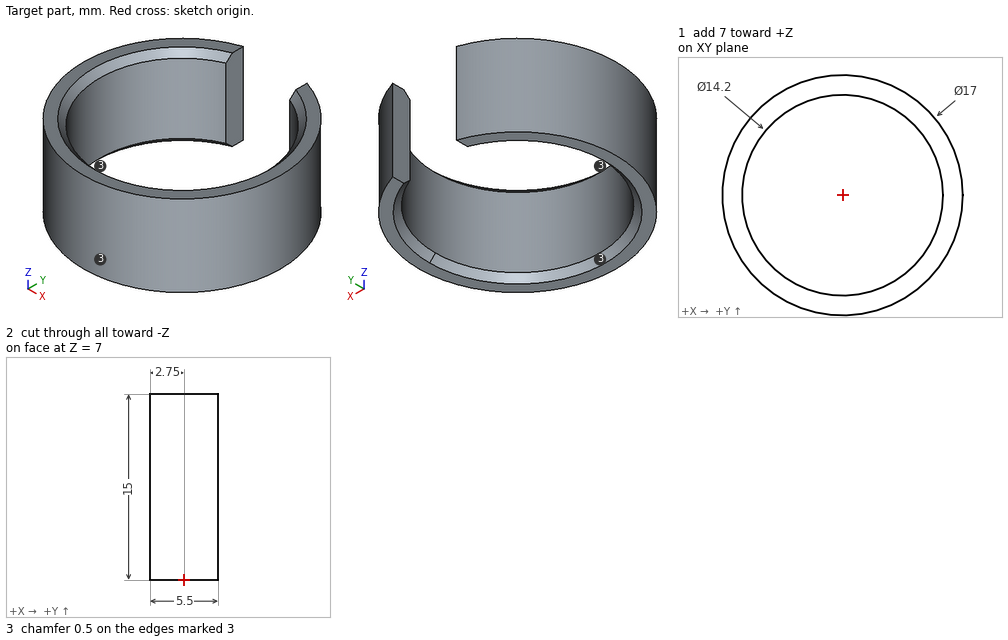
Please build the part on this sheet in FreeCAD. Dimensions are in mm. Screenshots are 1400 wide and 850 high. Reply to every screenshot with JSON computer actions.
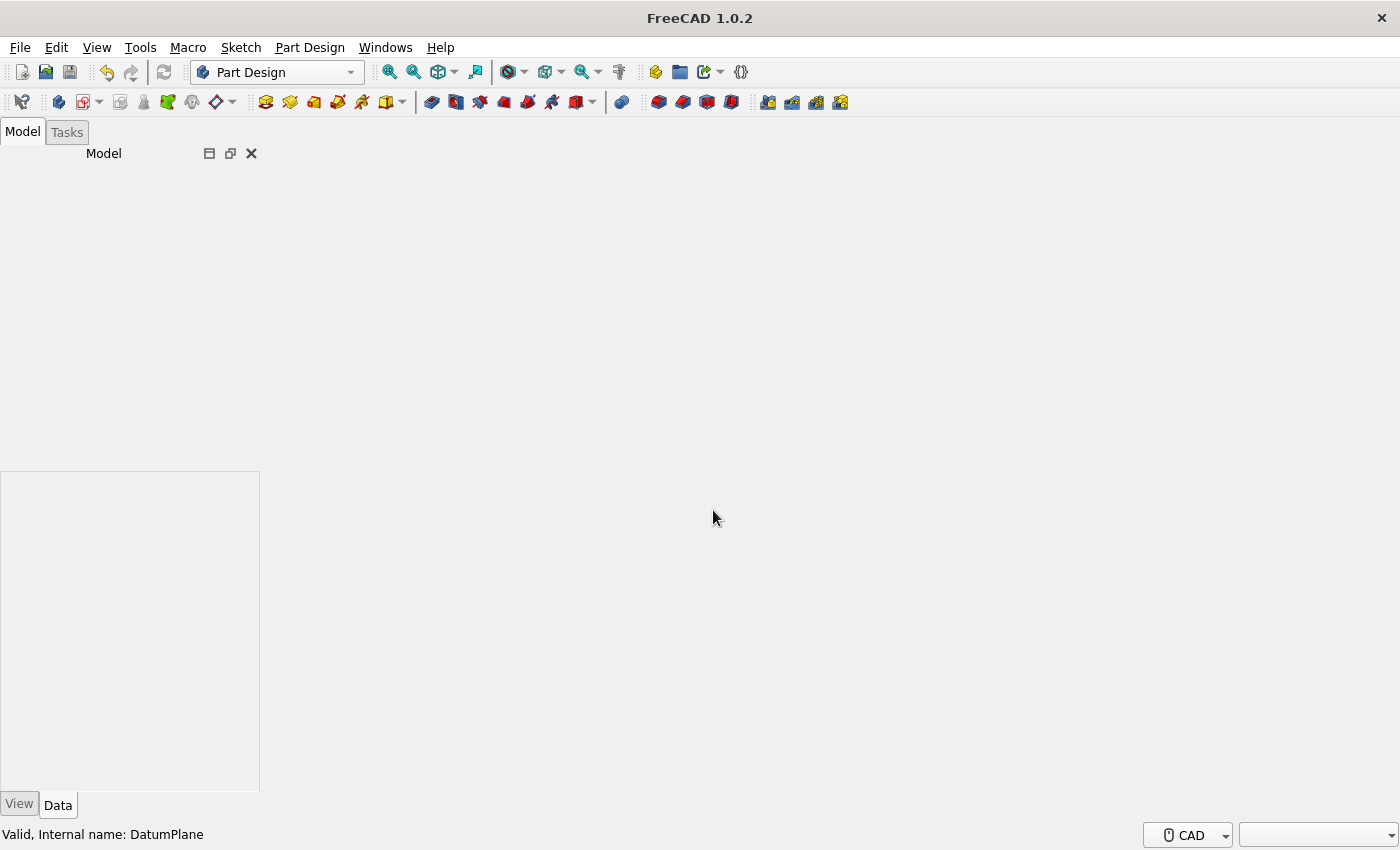
{"action": "left_click", "coordinate": [22, 72]}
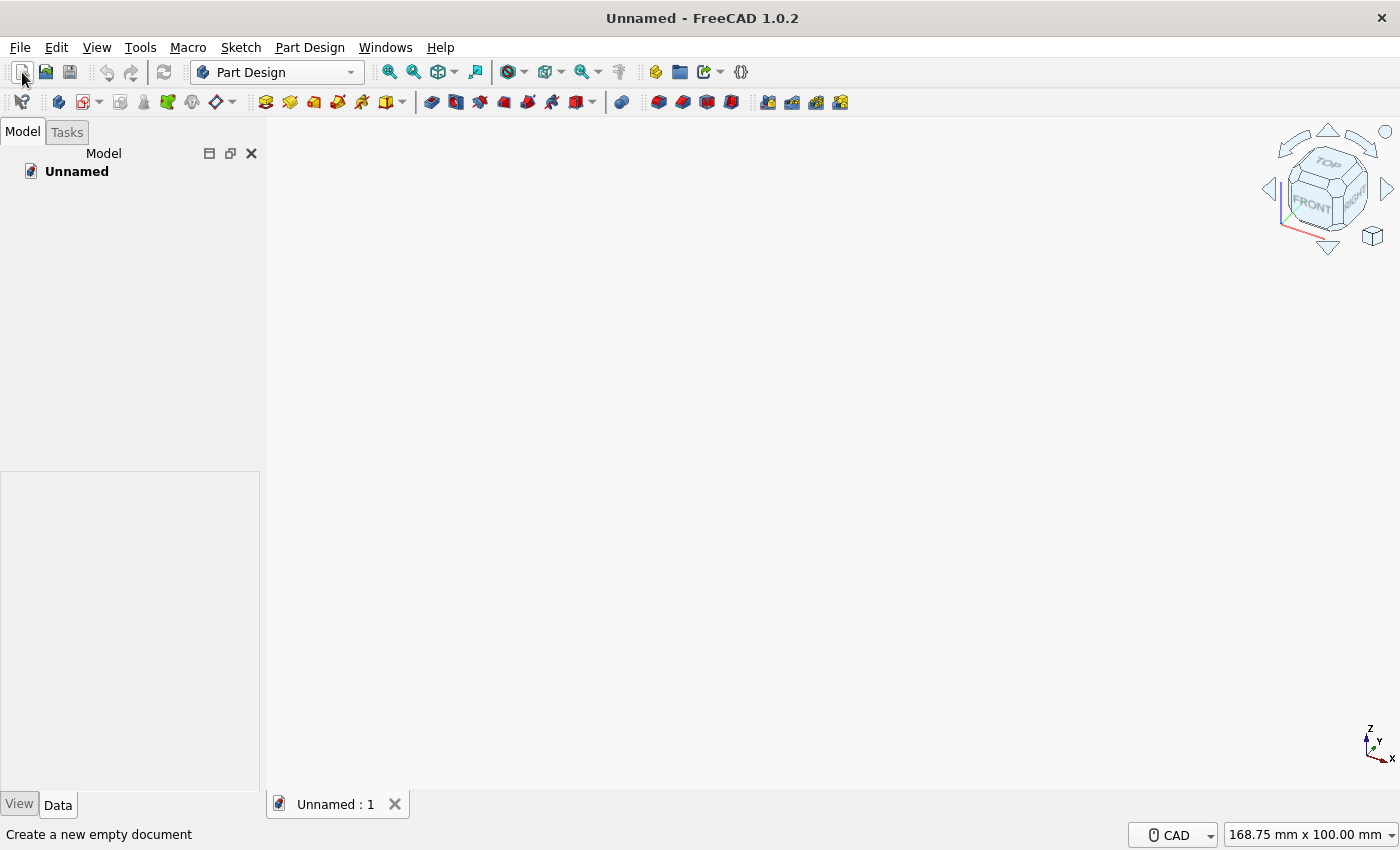
{"action": "left_click", "coordinate": [84, 102]}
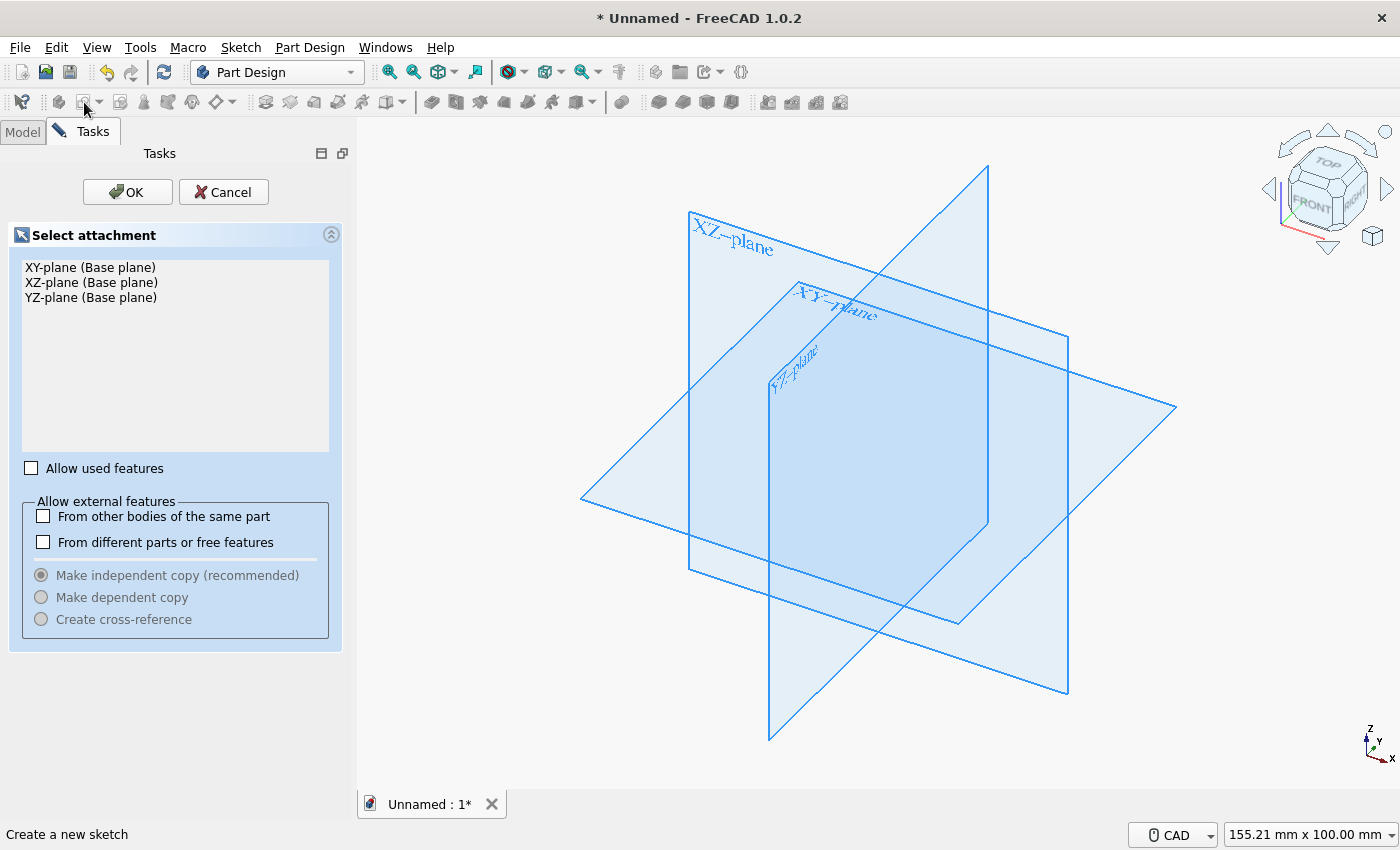
{"action": "left_click", "coordinate": [82, 268]}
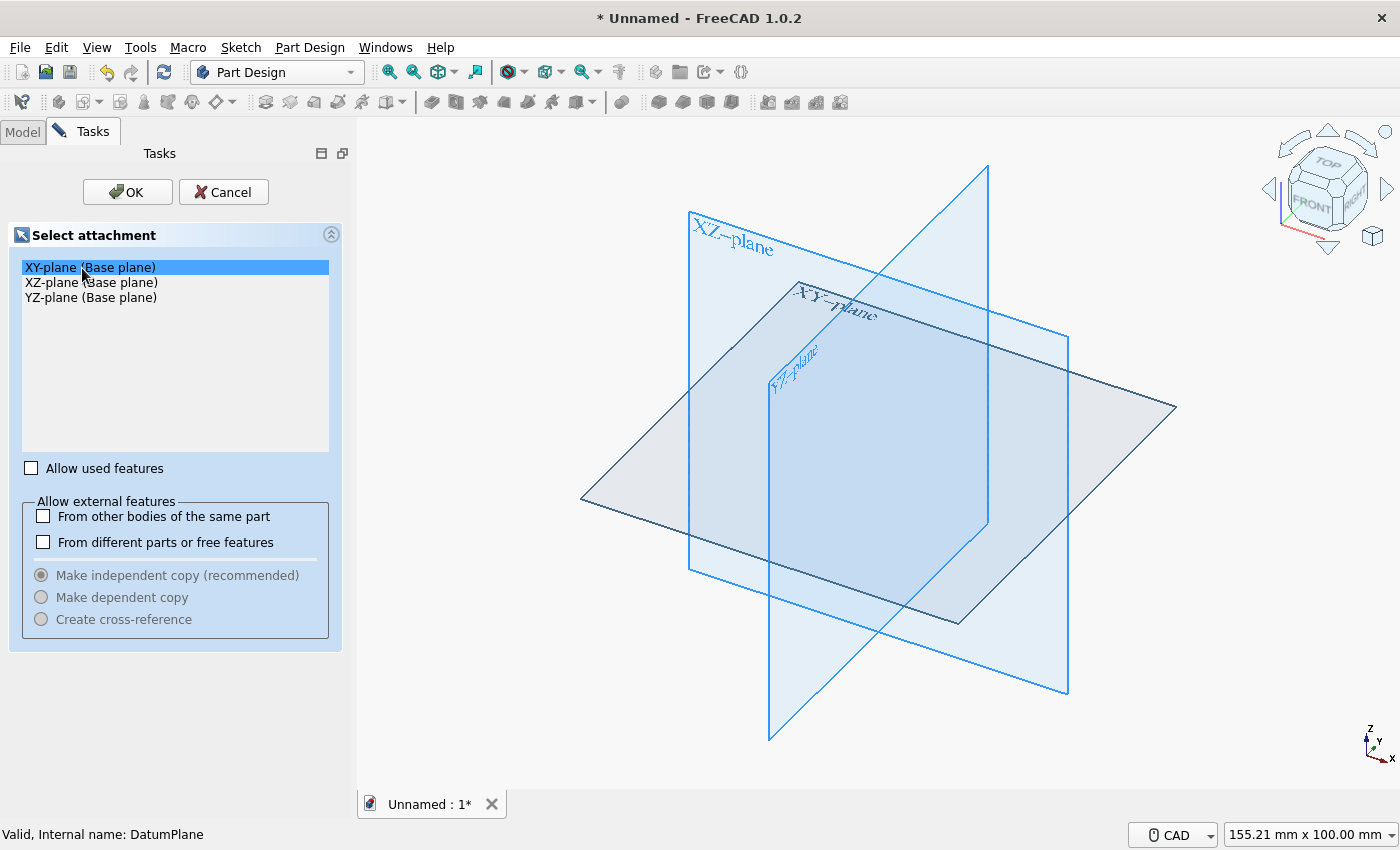
{"action": "left_click", "coordinate": [128, 192]}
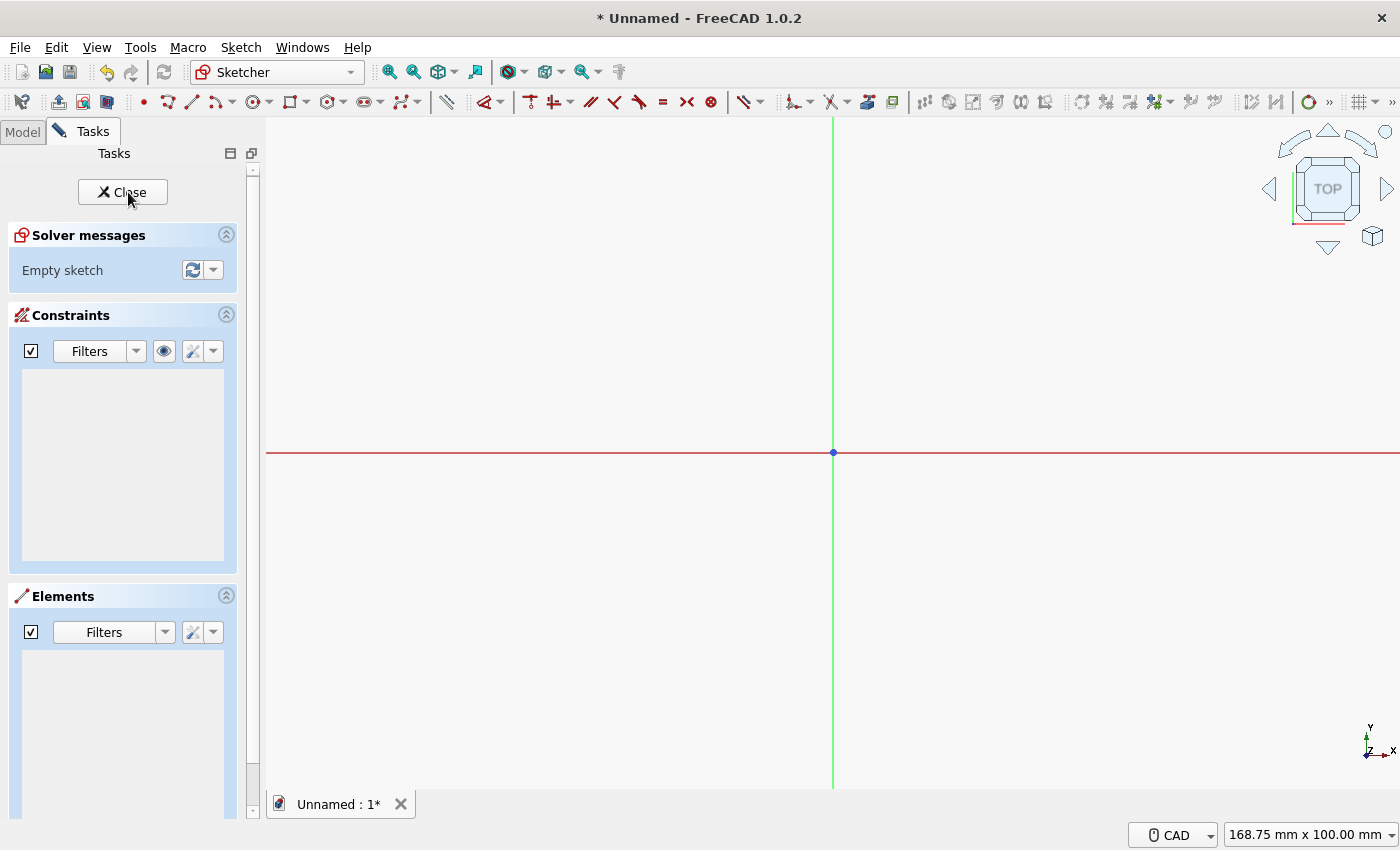
{"action": "scroll", "coordinate": [855, 453], "scroll_direction": "up", "scroll_amount": 7}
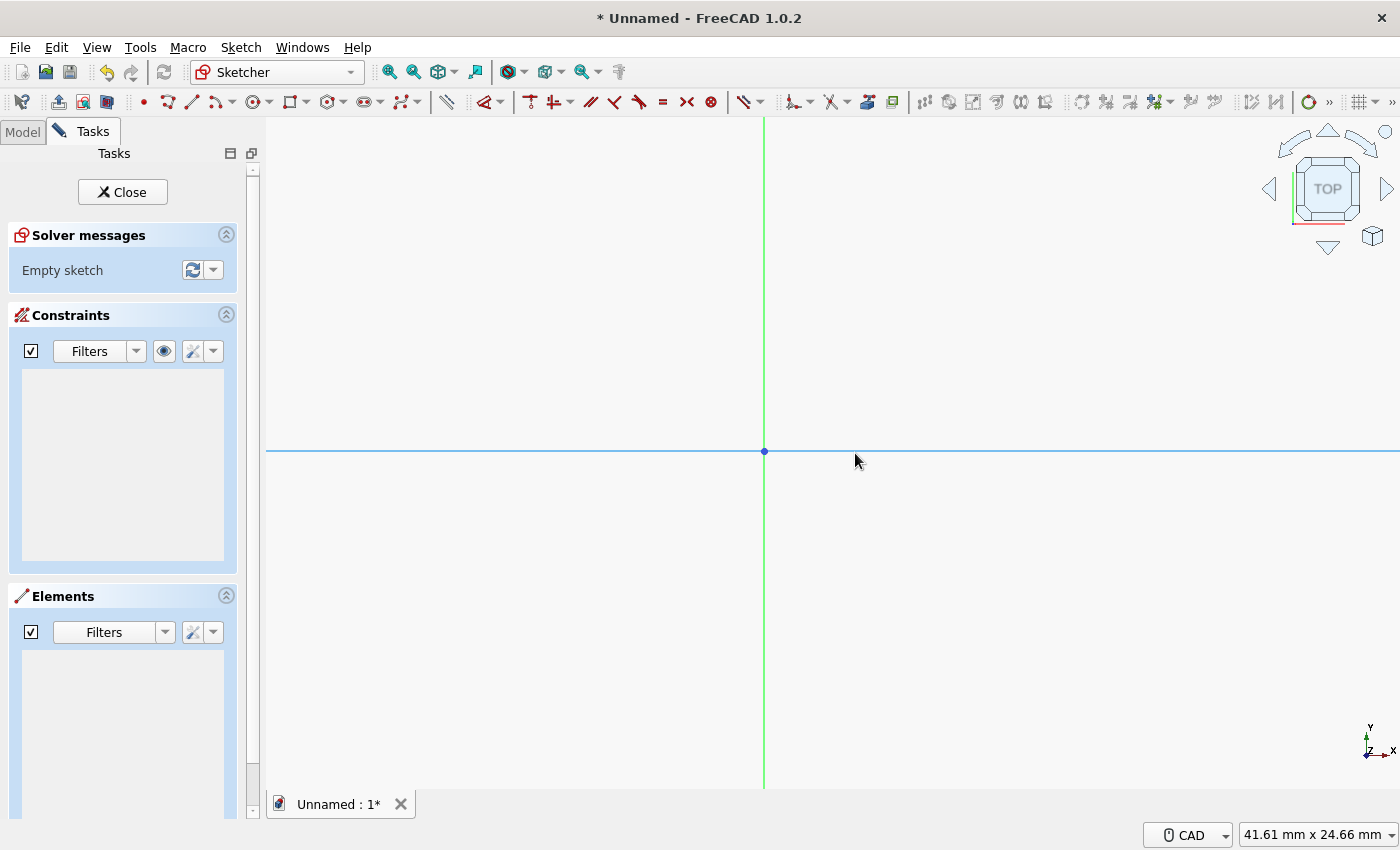
{"action": "left_click", "coordinate": [254, 102]}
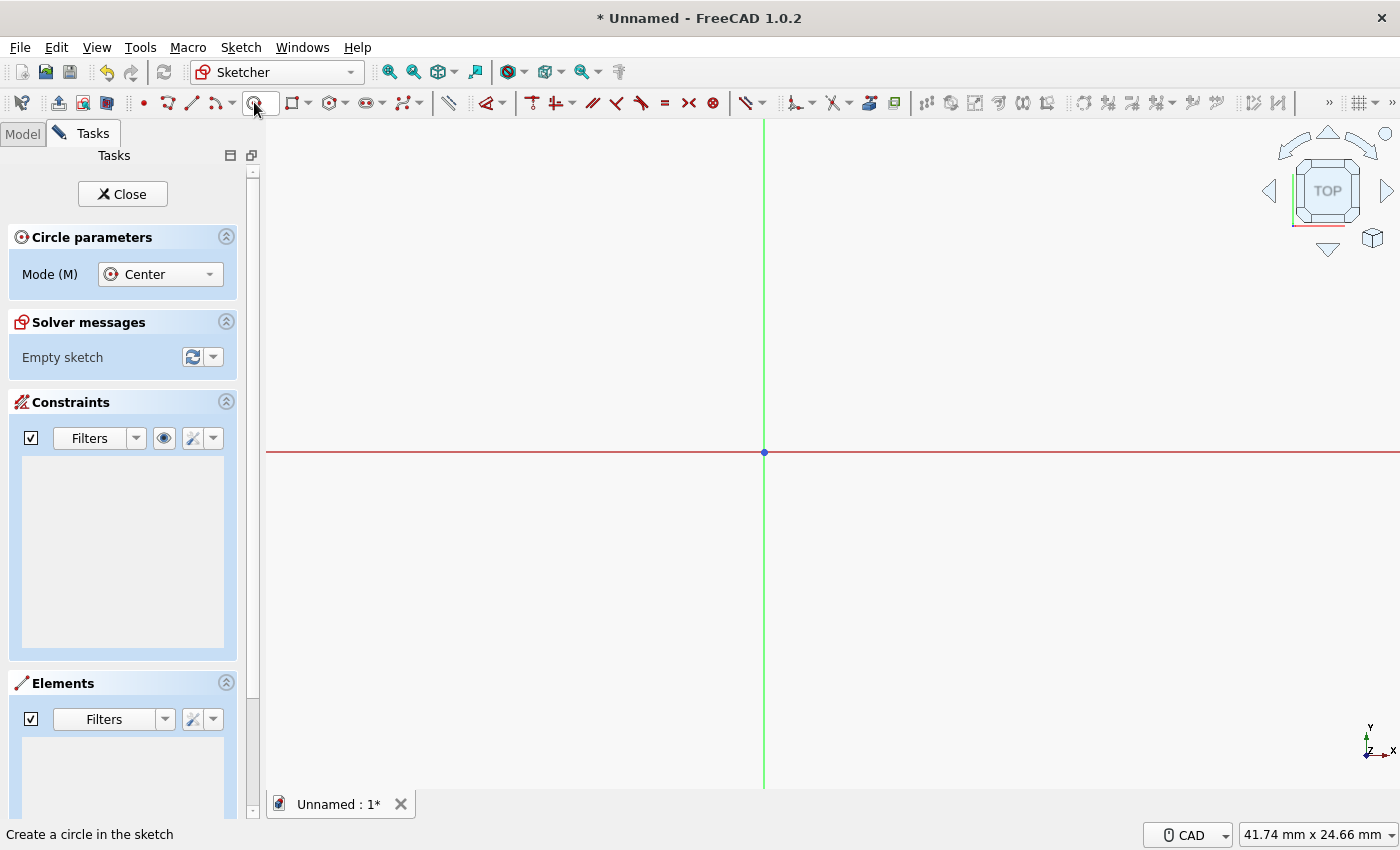
{"action": "left_click", "coordinate": [764, 452]}
{"action": "mouse_move", "coordinate": [928, 289]}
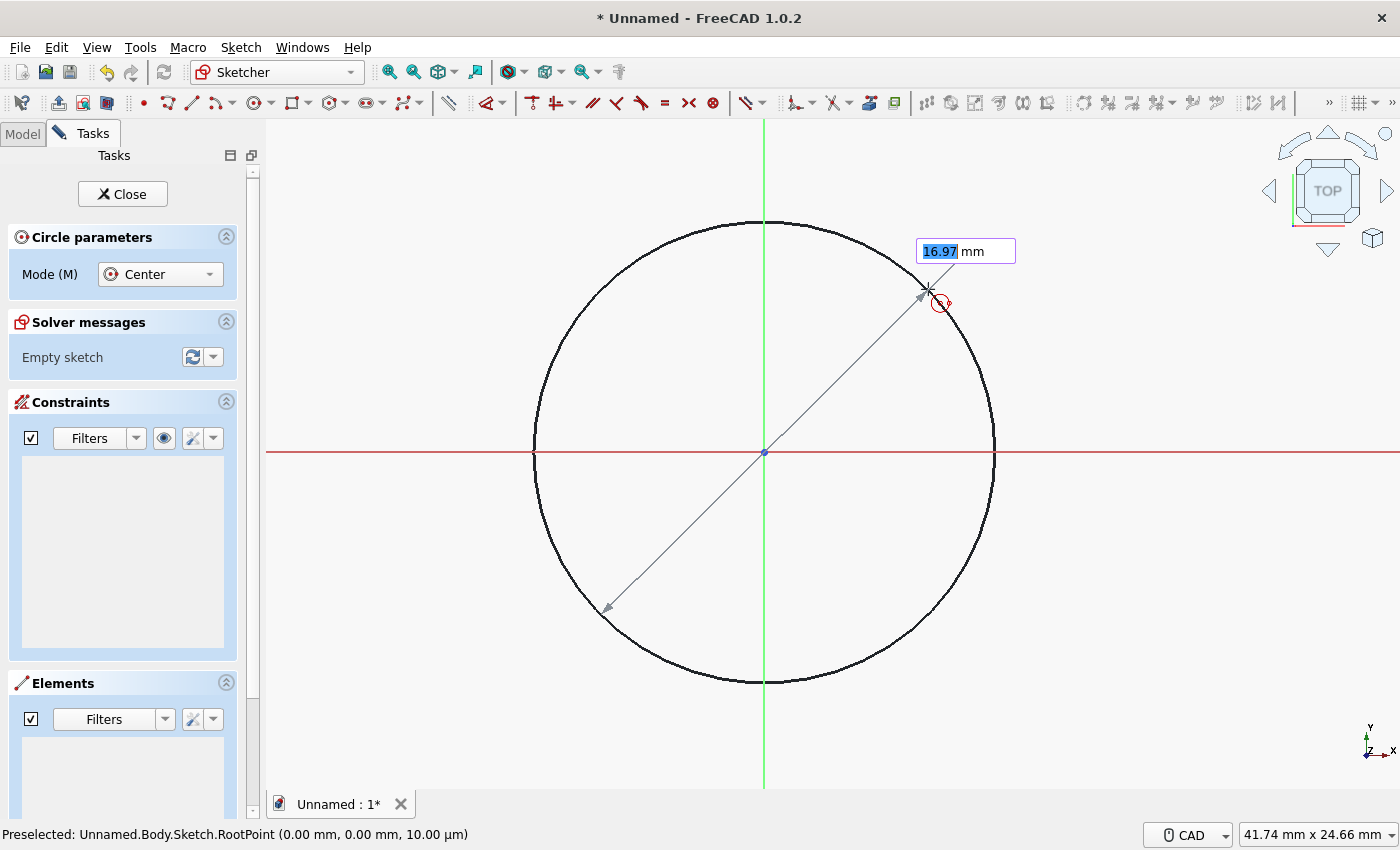
{"action": "type", "text": "17"}
{"action": "key", "text": "Return"}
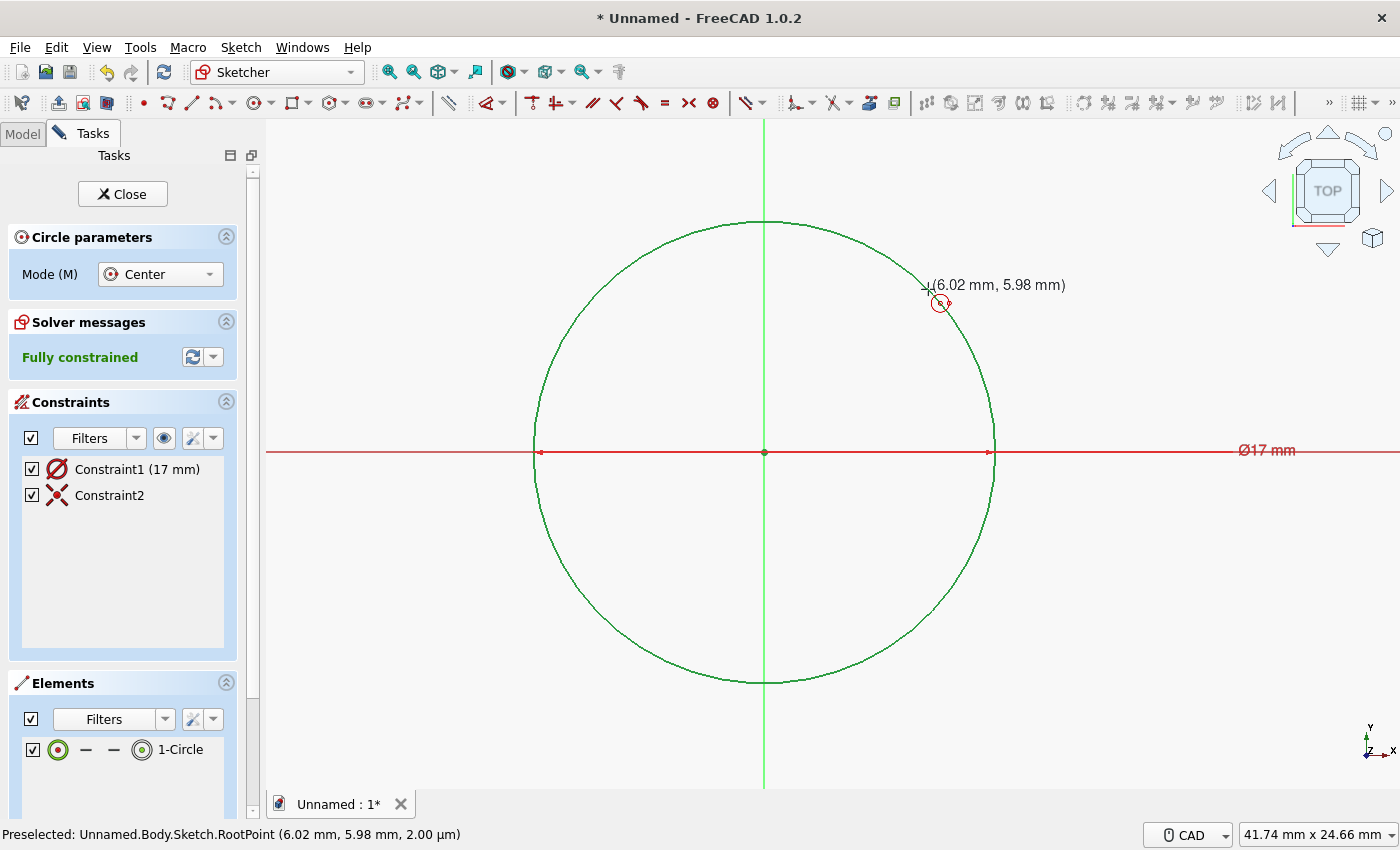
{"action": "left_click", "coordinate": [764, 452]}
{"action": "mouse_move", "coordinate": [901, 316]}